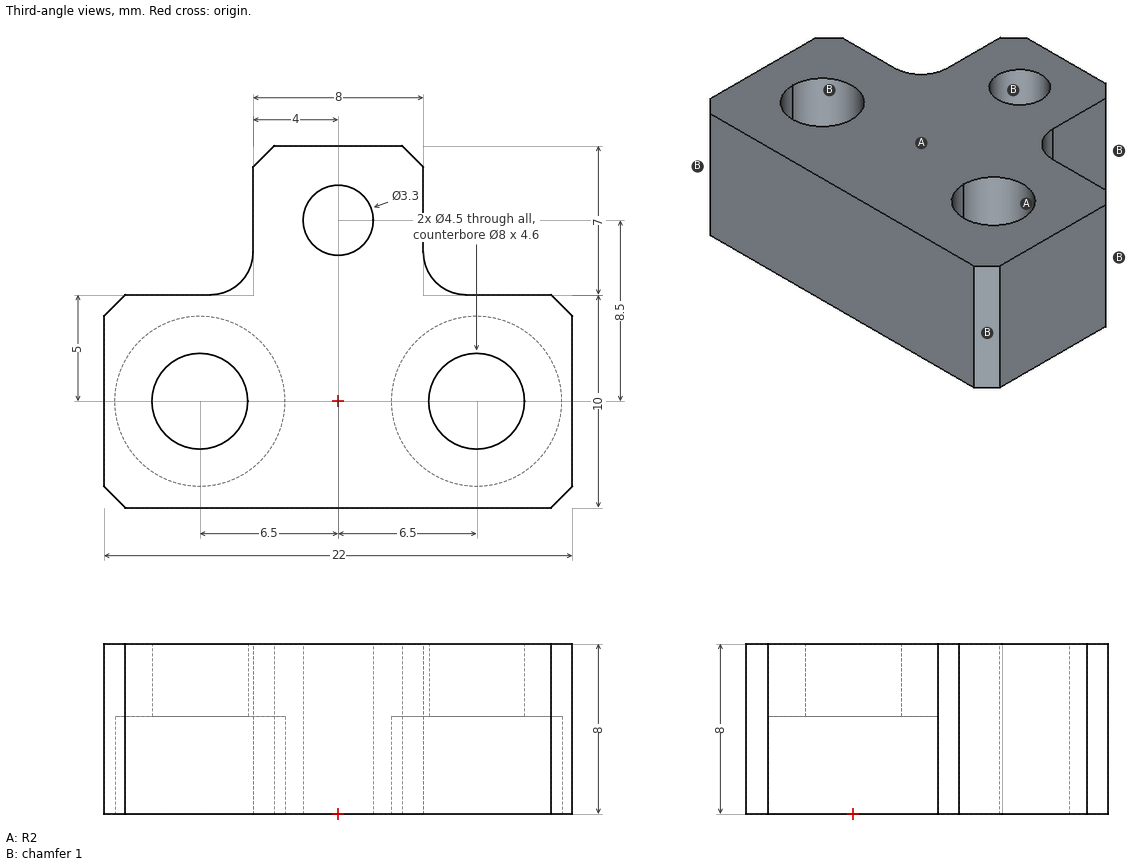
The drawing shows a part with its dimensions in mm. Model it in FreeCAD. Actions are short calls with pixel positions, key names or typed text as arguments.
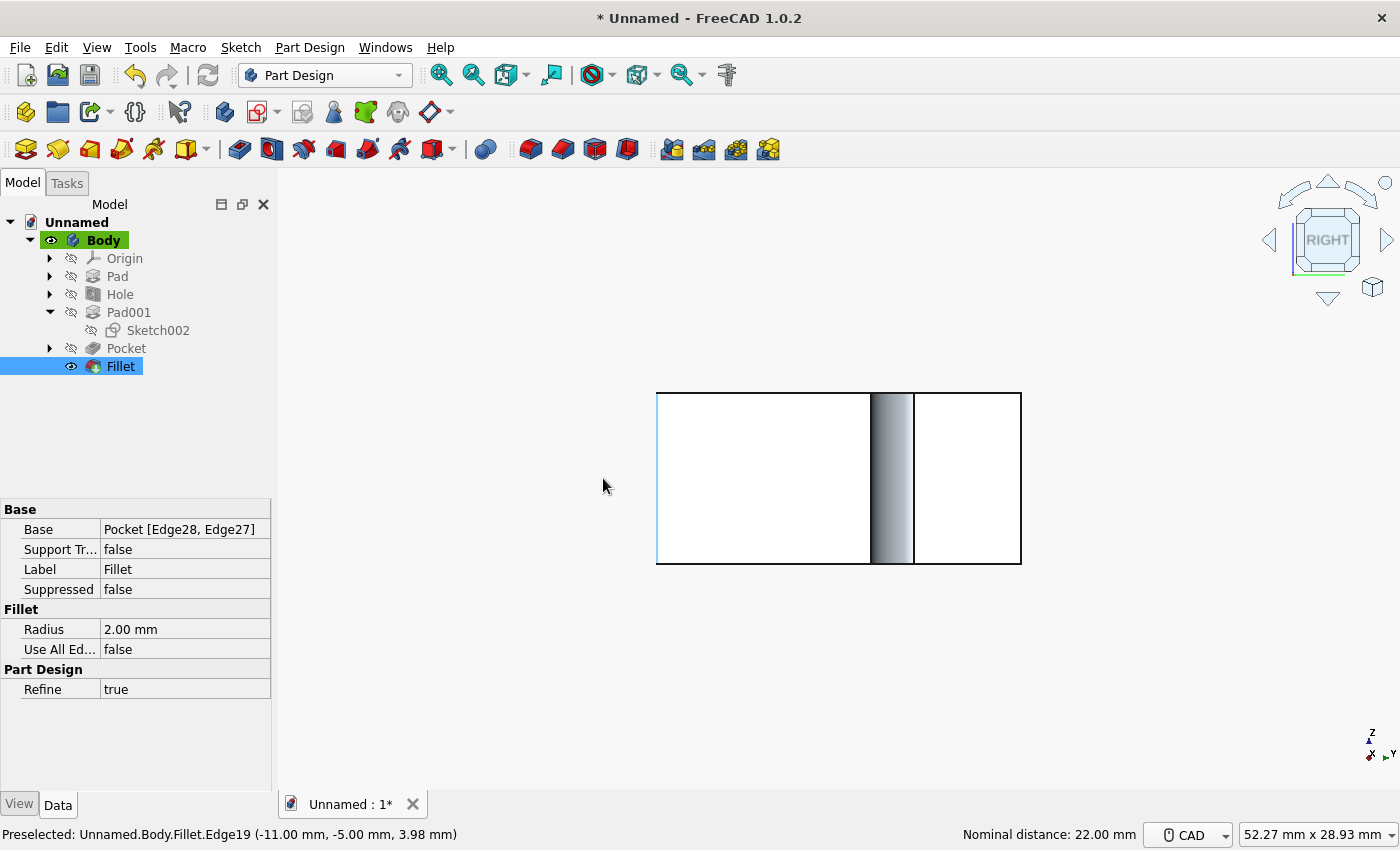
click(442, 76)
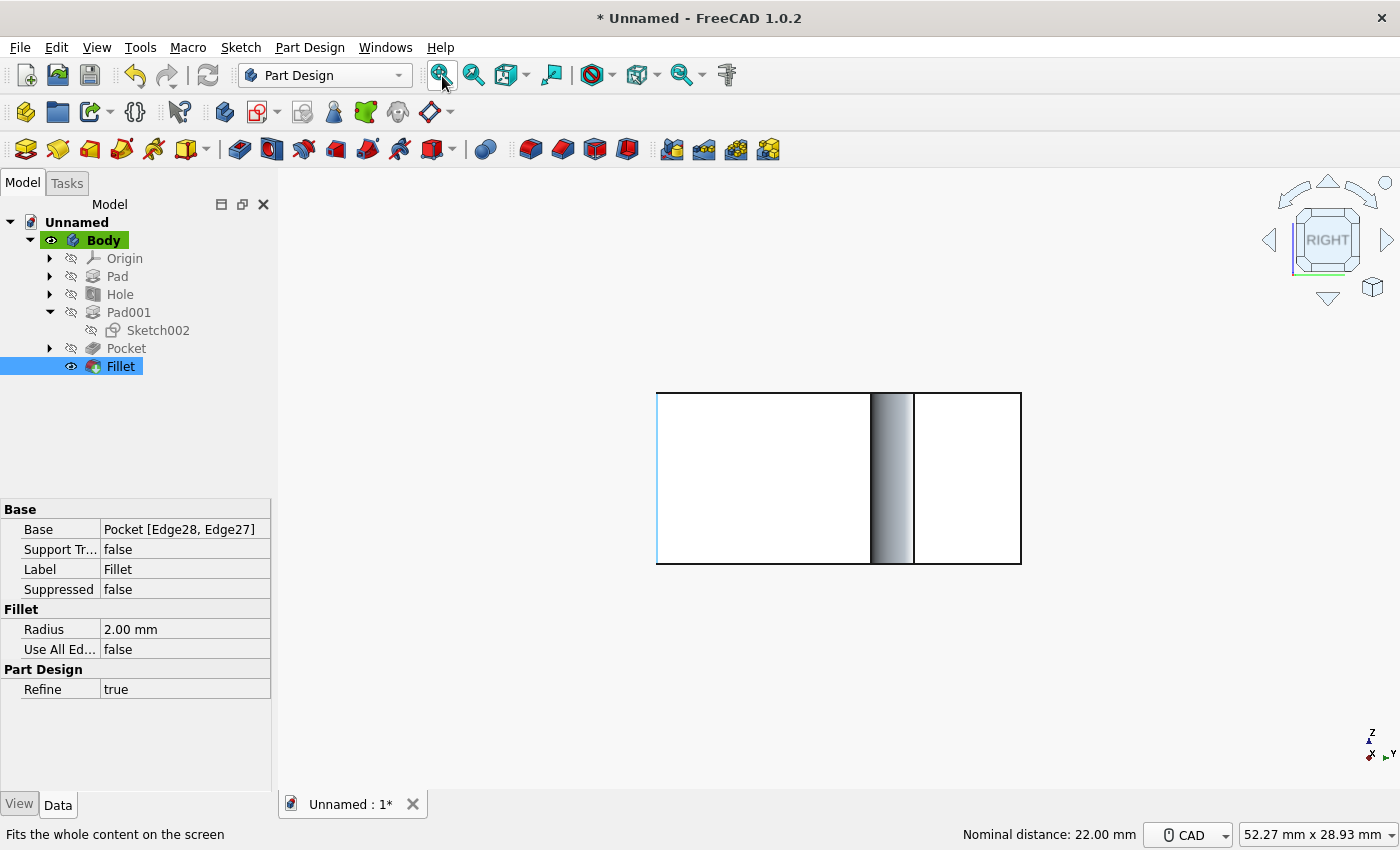
click(1021, 477, ctrl)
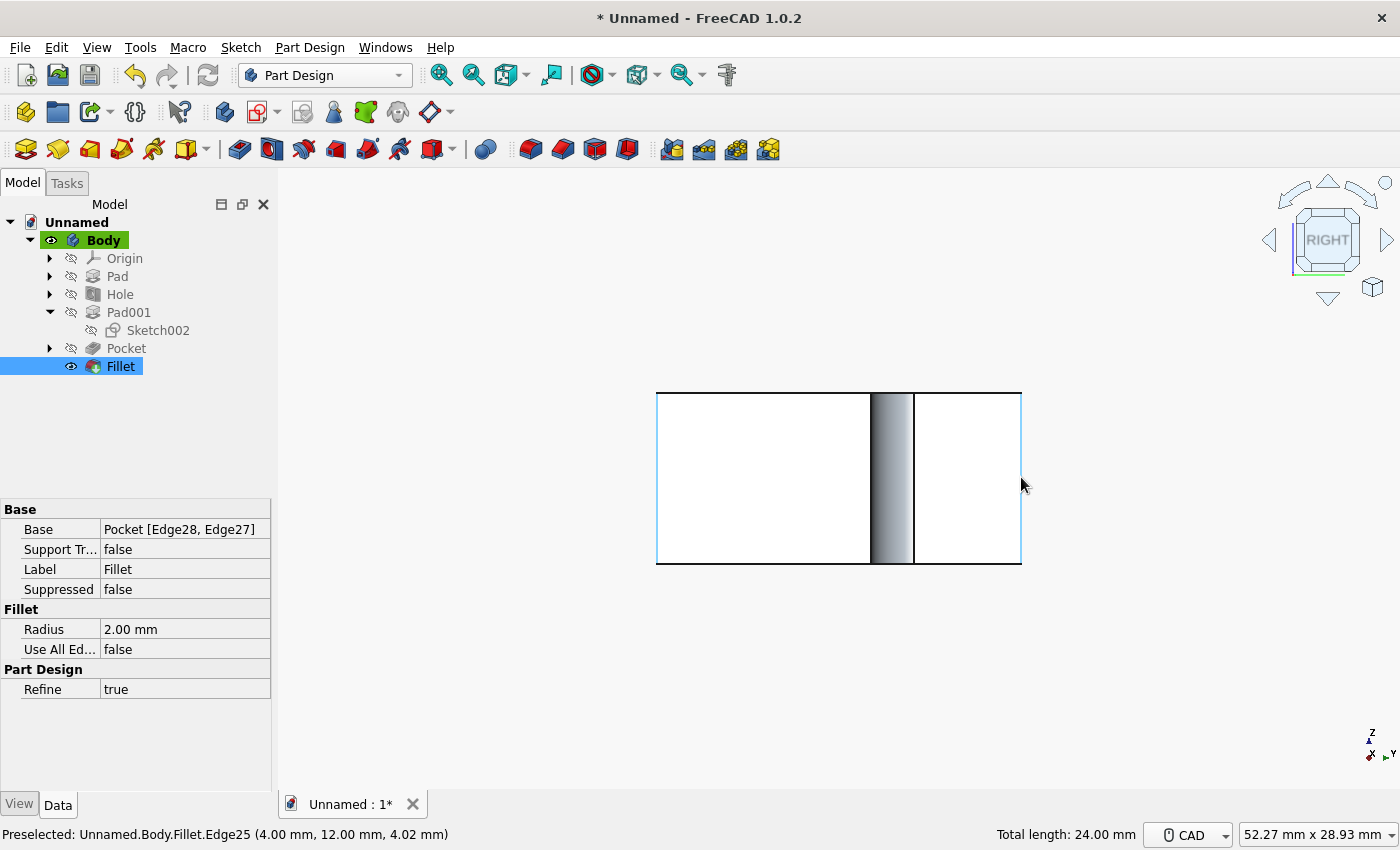
click(871, 477, ctrl)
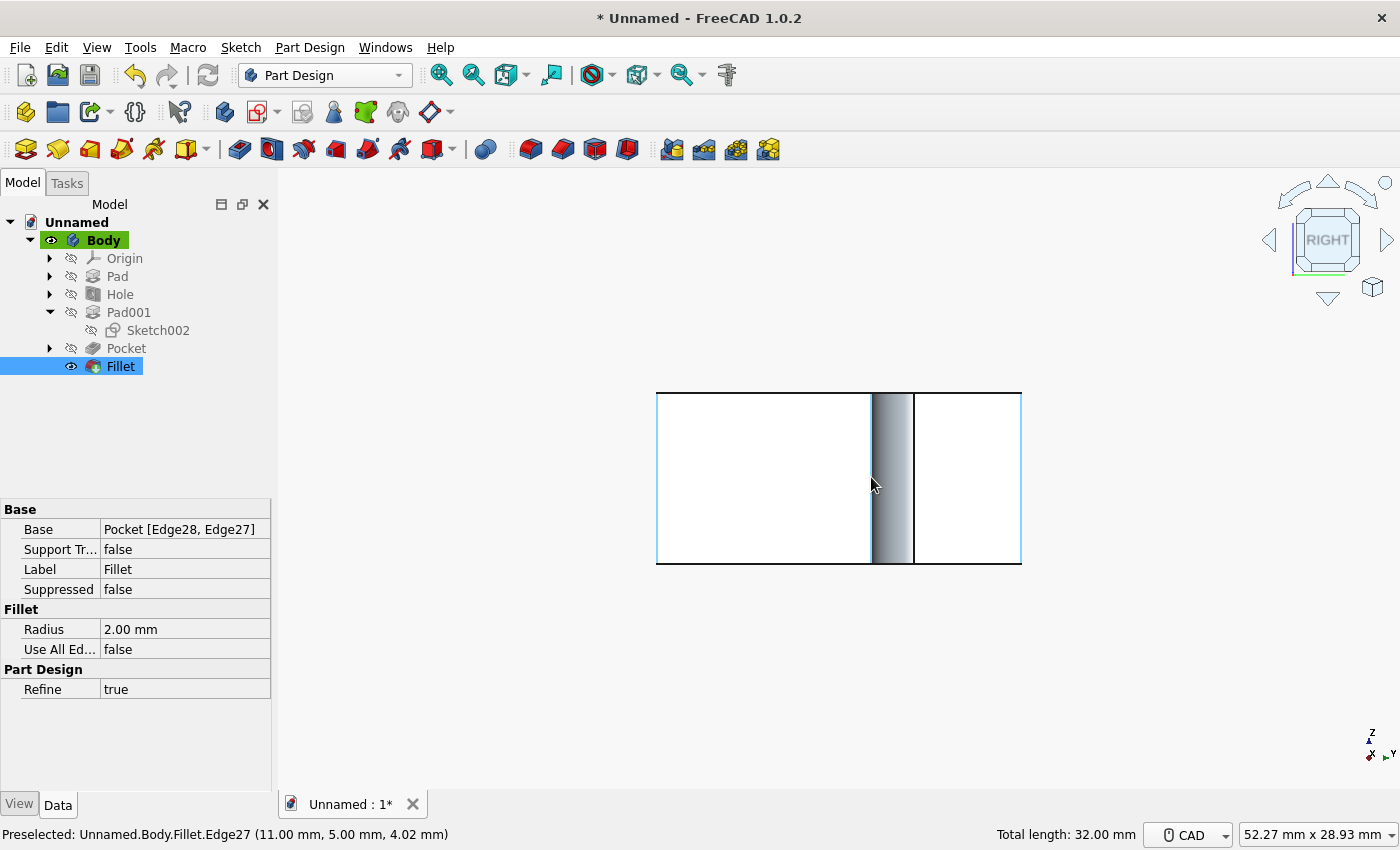
key(5)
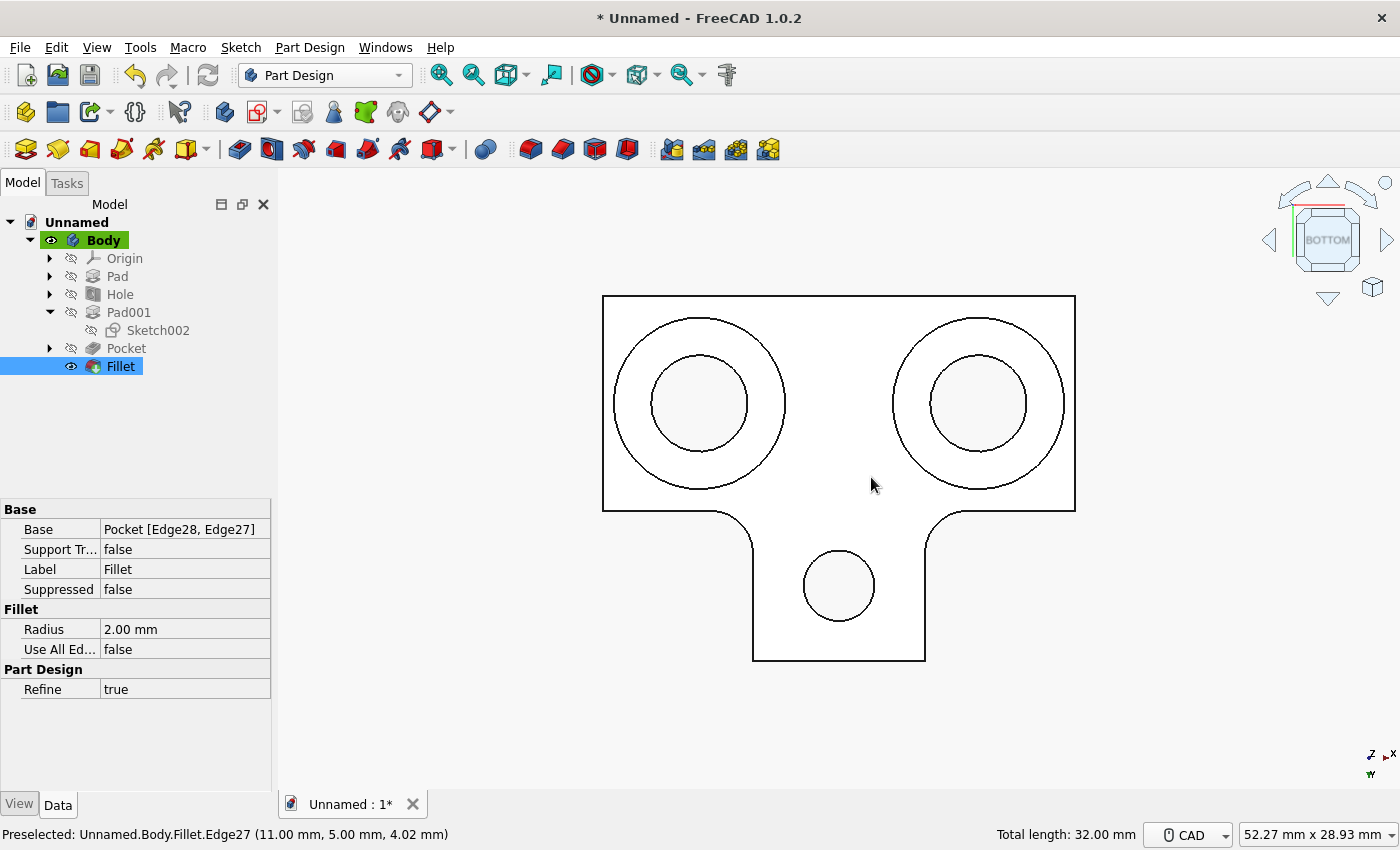
key(4)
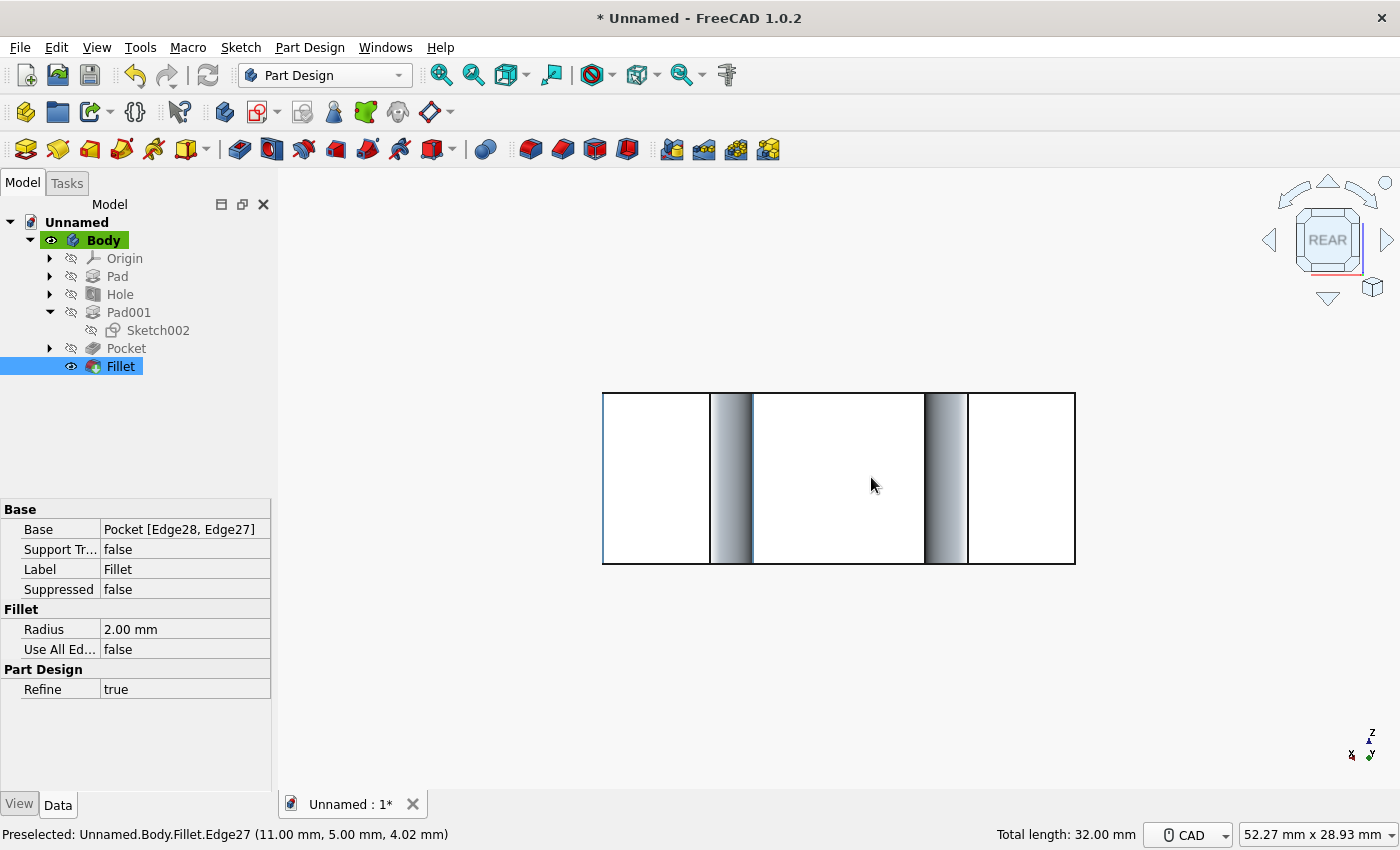
click(442, 76)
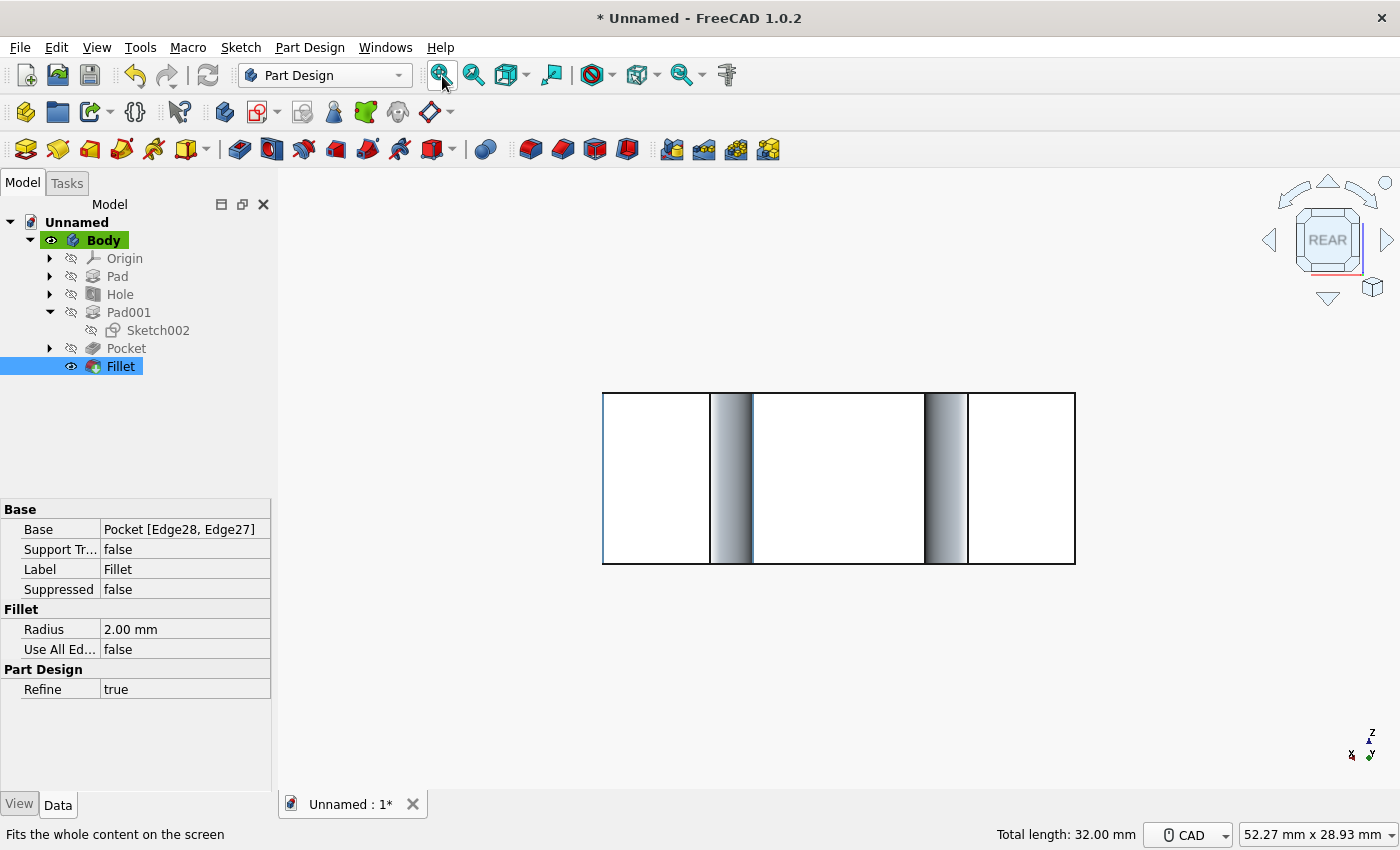
click(925, 478, ctrl)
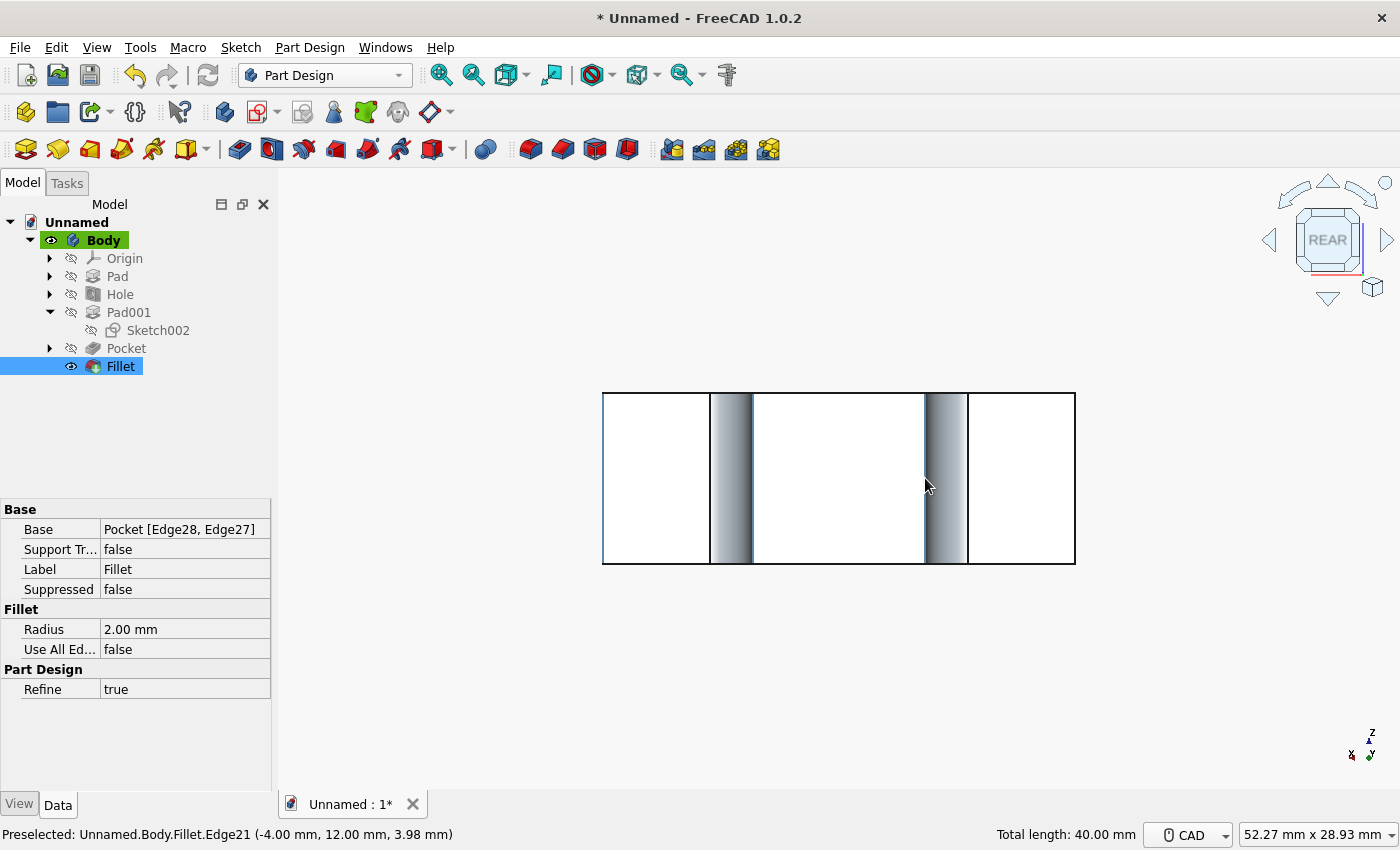
click(1075, 478, ctrl)